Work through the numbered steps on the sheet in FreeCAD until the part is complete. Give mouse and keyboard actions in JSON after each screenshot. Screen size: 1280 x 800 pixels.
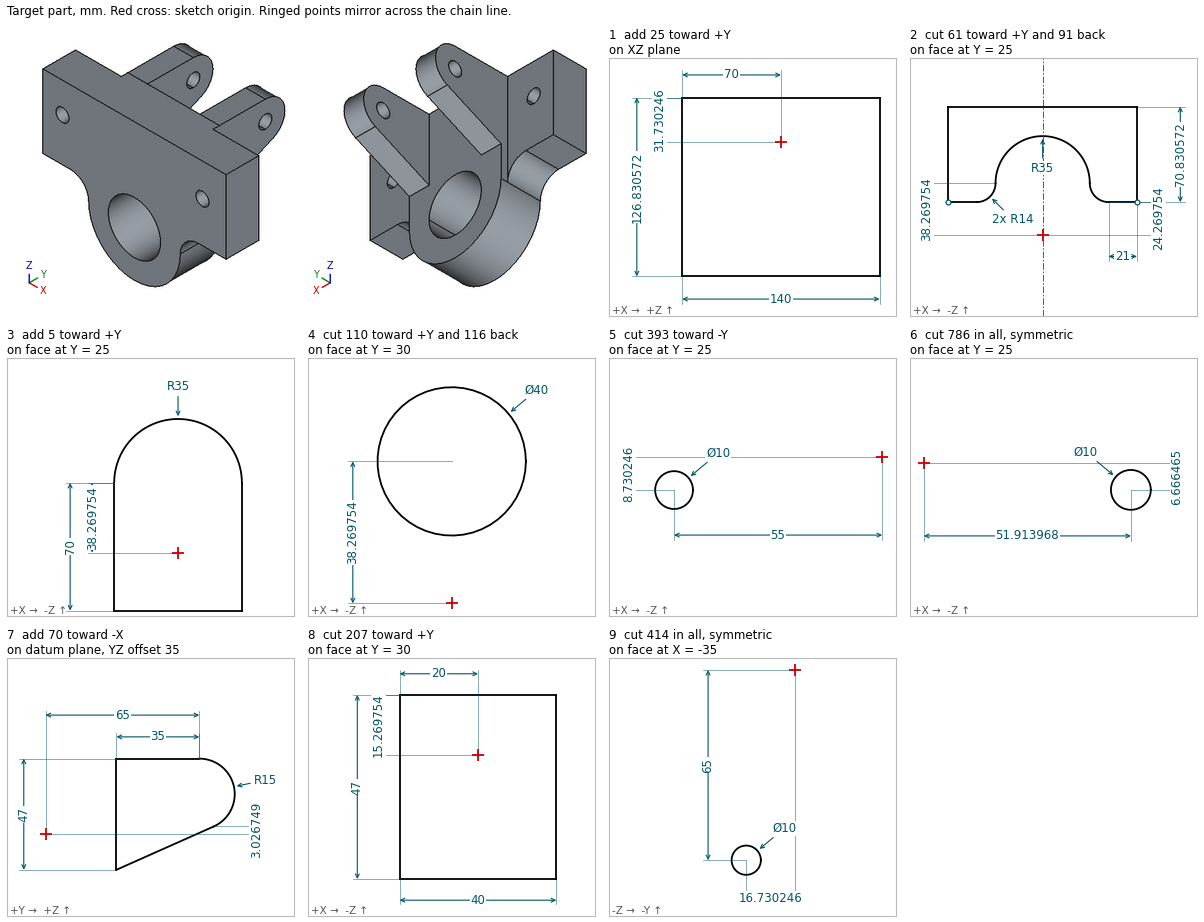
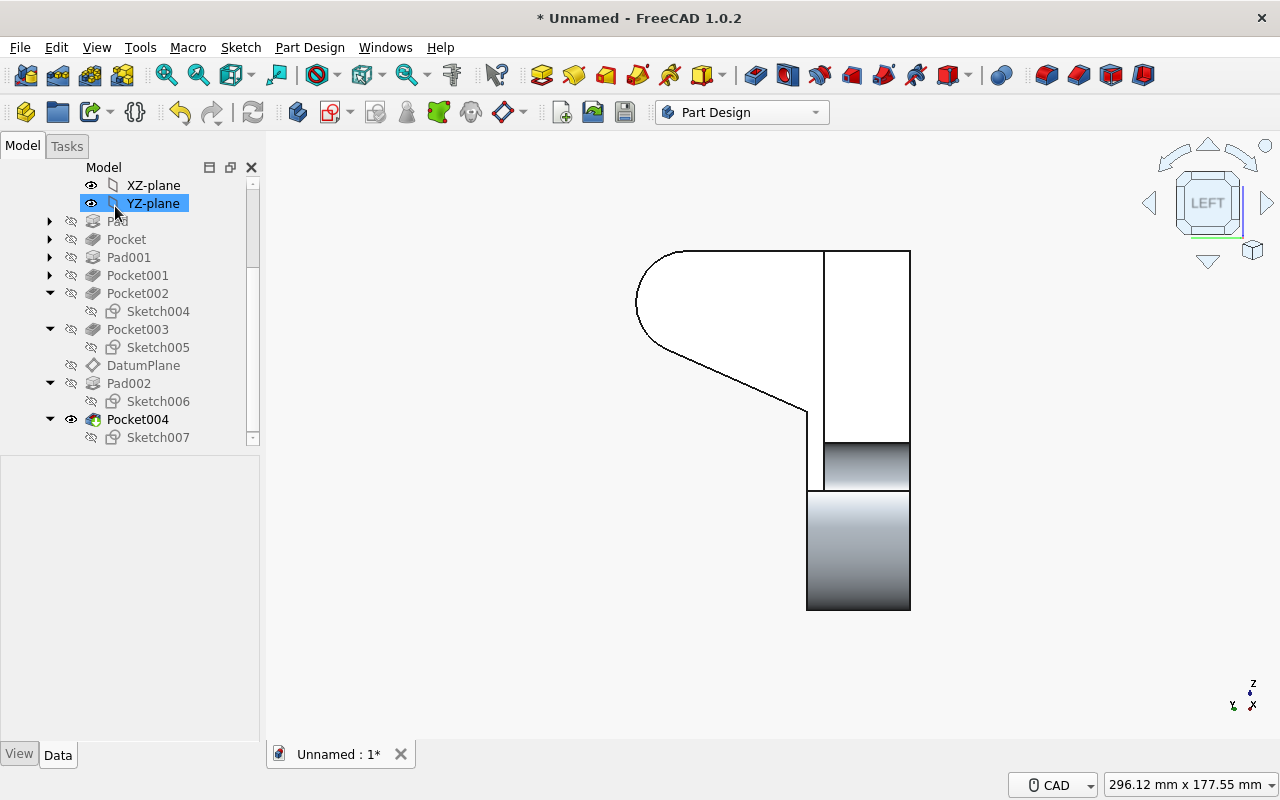
{"action": "left_click", "coordinate": [730, 301]}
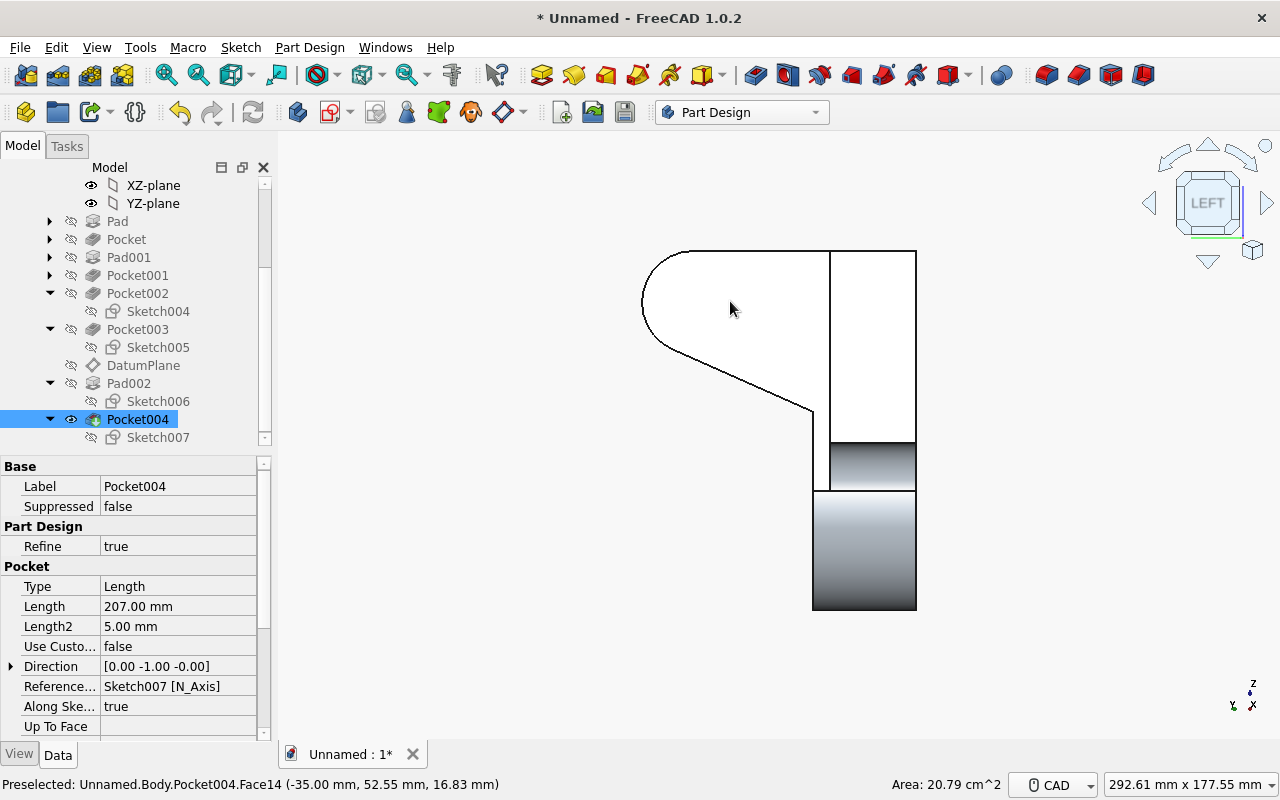
{"action": "left_click", "coordinate": [330, 112]}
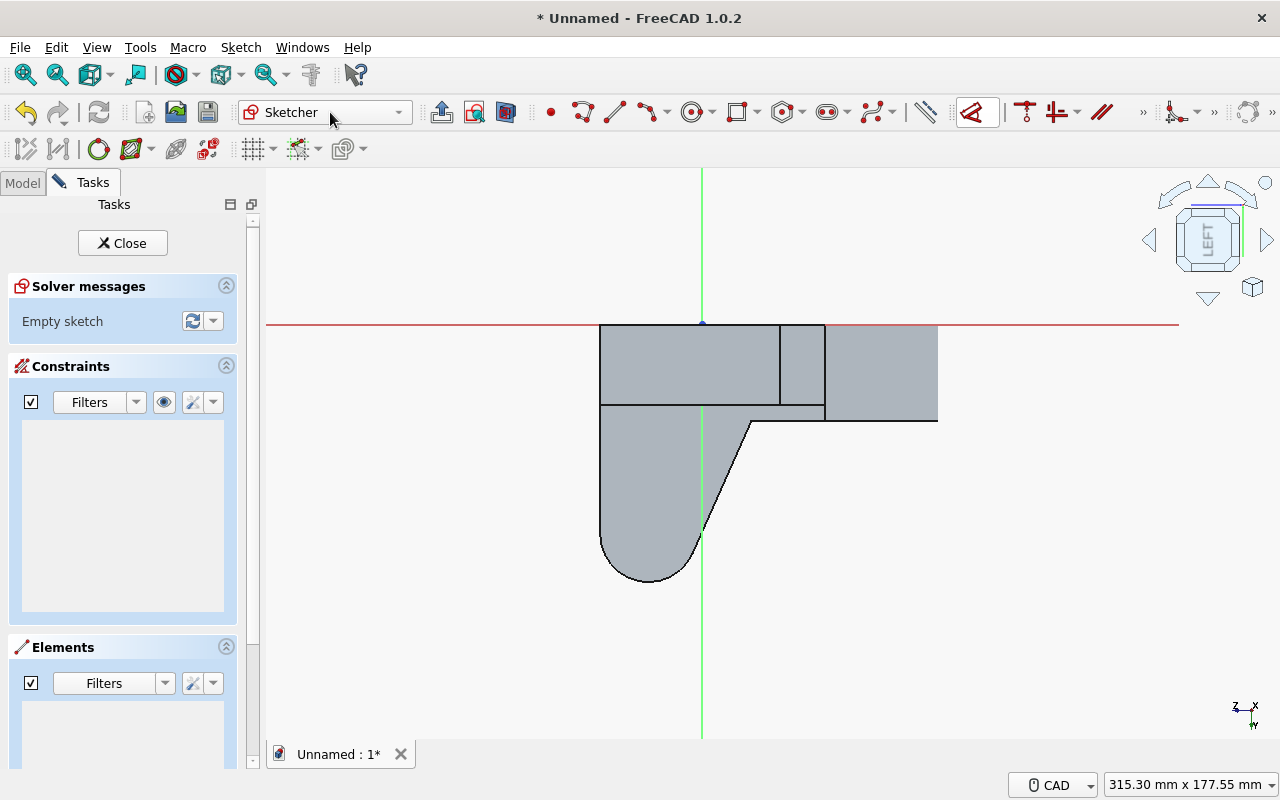
{"action": "left_click", "coordinate": [506, 112]}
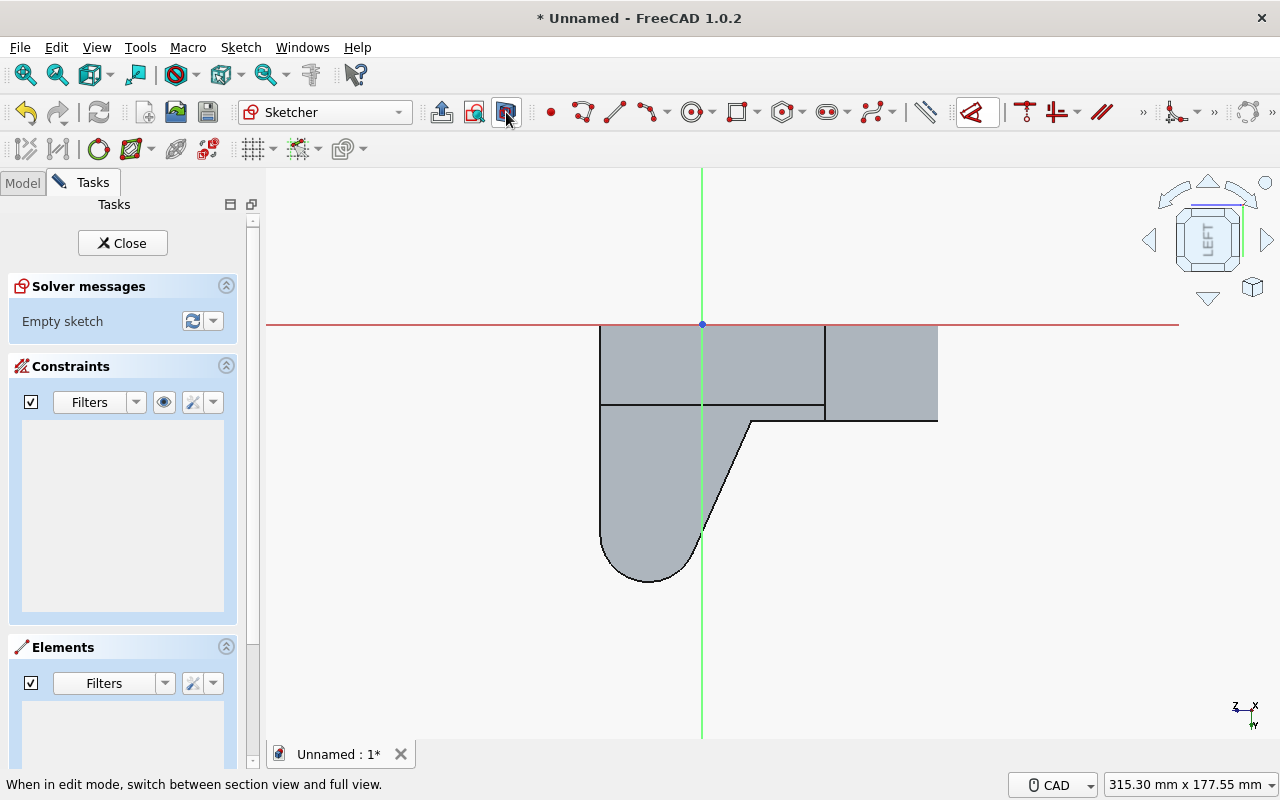
{"action": "scroll", "coordinate": [643, 542], "scroll_direction": "up", "scroll_amount": 12}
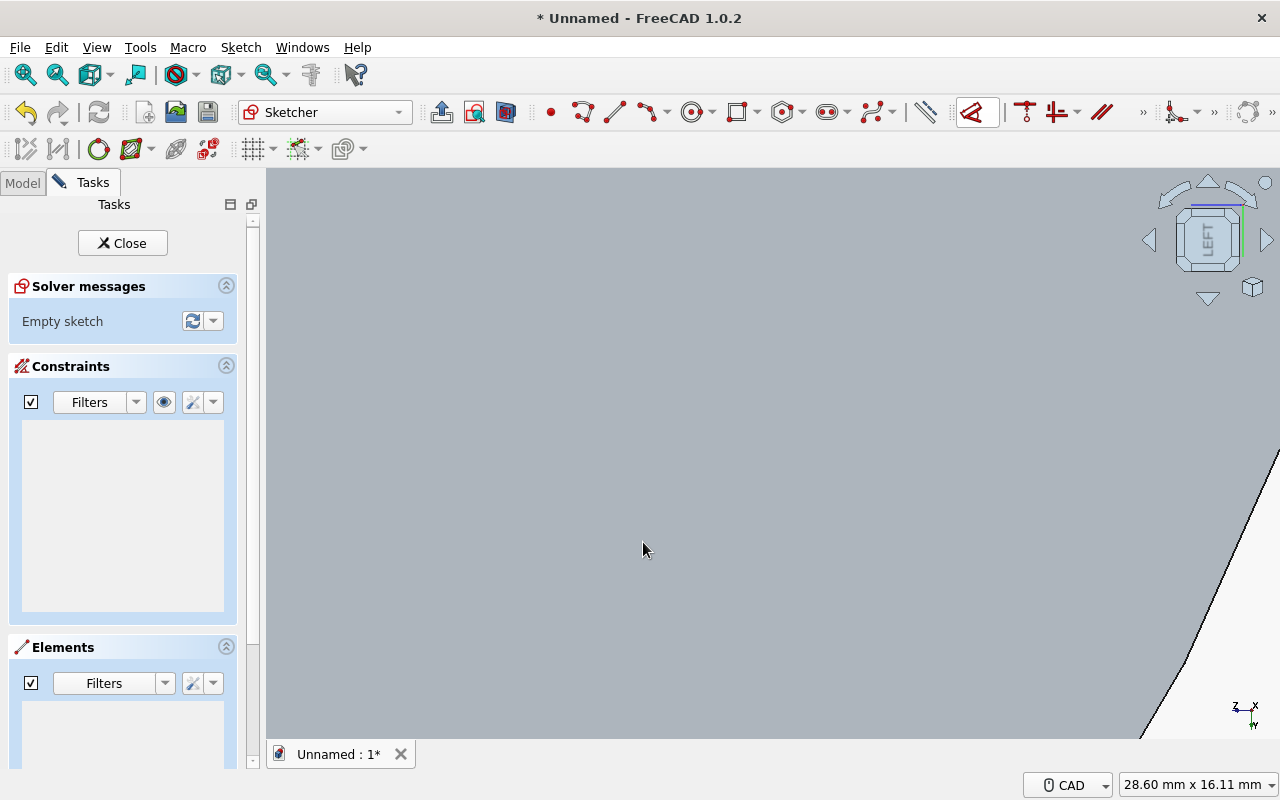
{"action": "left_click", "coordinate": [692, 112]}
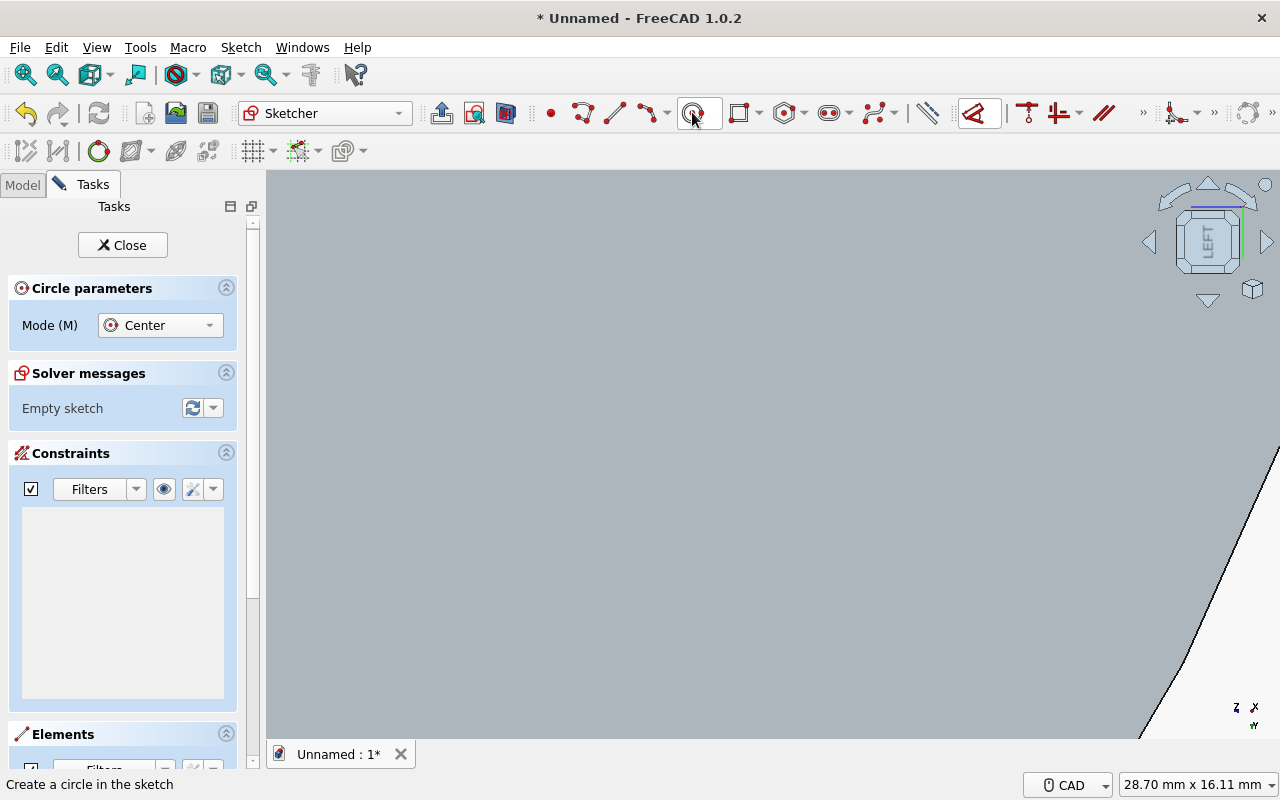
{"action": "left_click", "coordinate": [699, 447]}
{"action": "left_click", "coordinate": [824, 323]}
{"action": "key", "text": "Escape"}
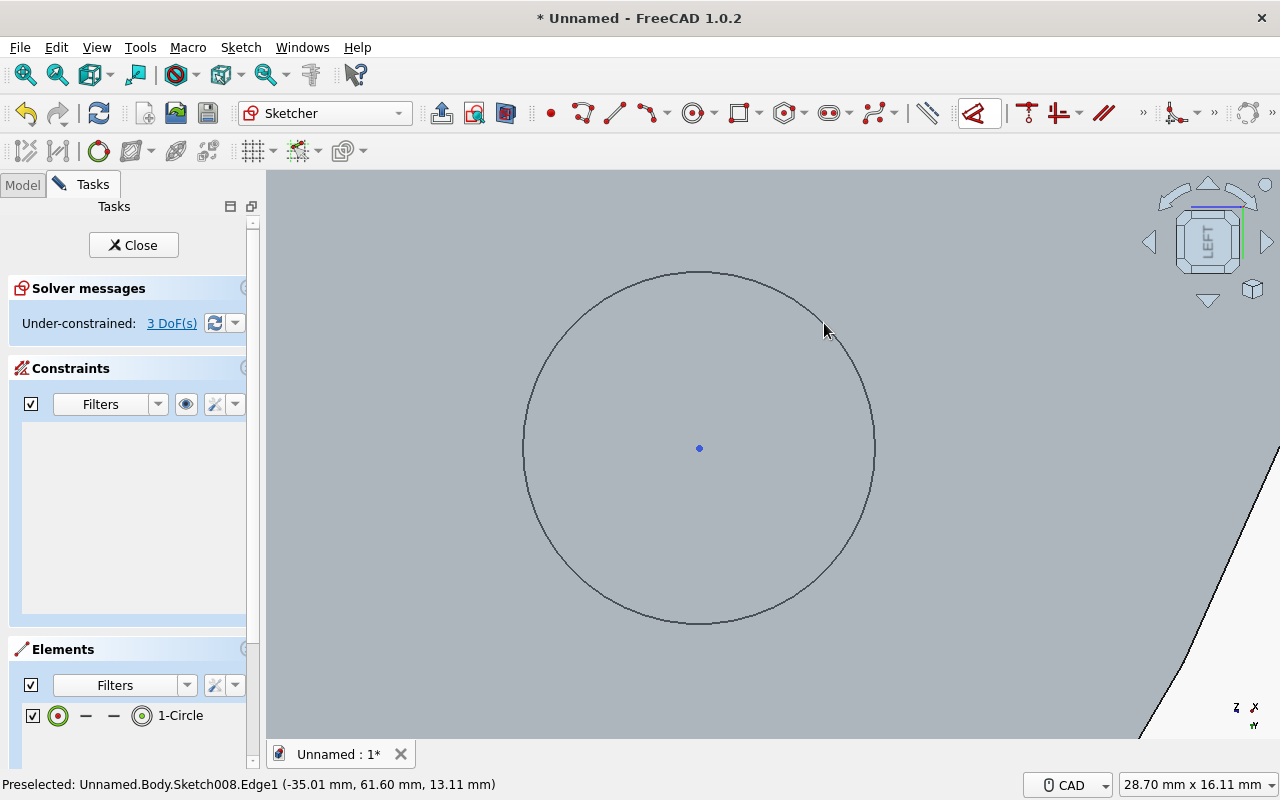
{"action": "left_click", "coordinate": [823, 323]}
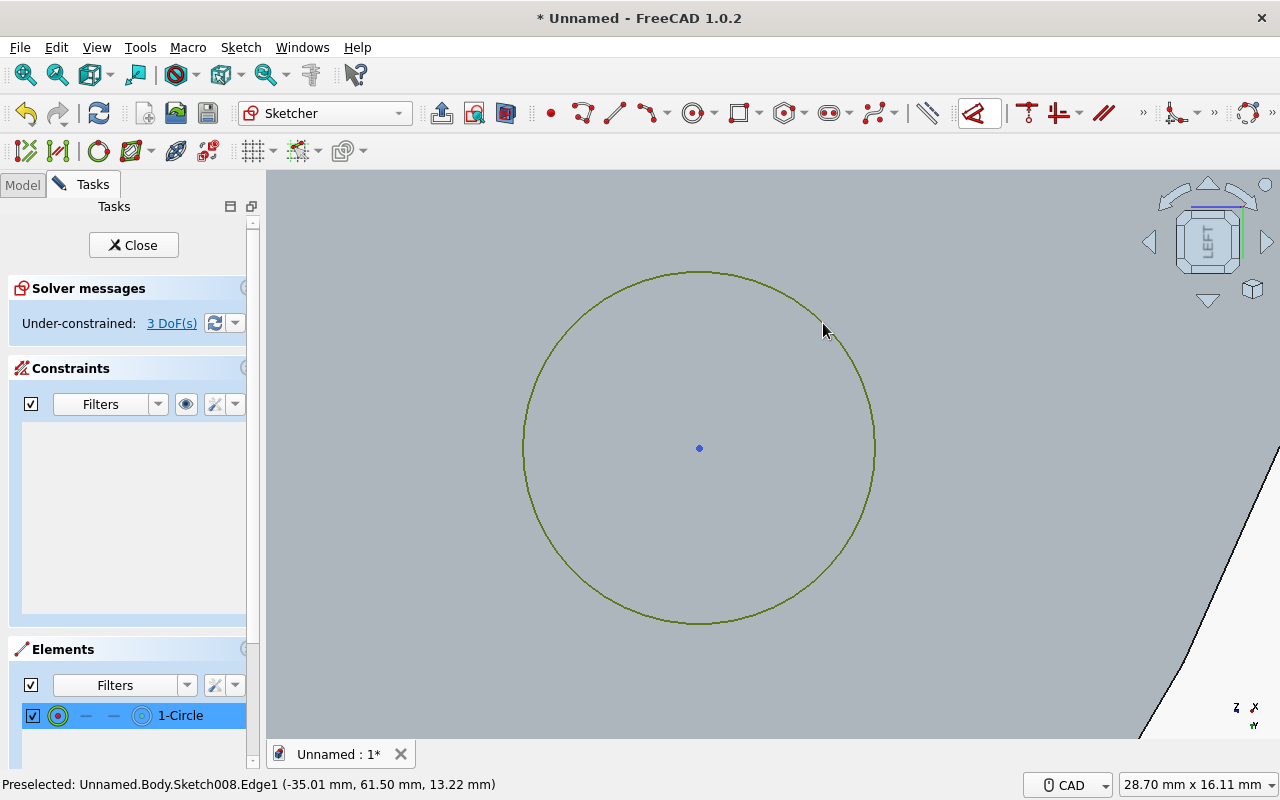
{"action": "left_click", "coordinate": [996, 114]}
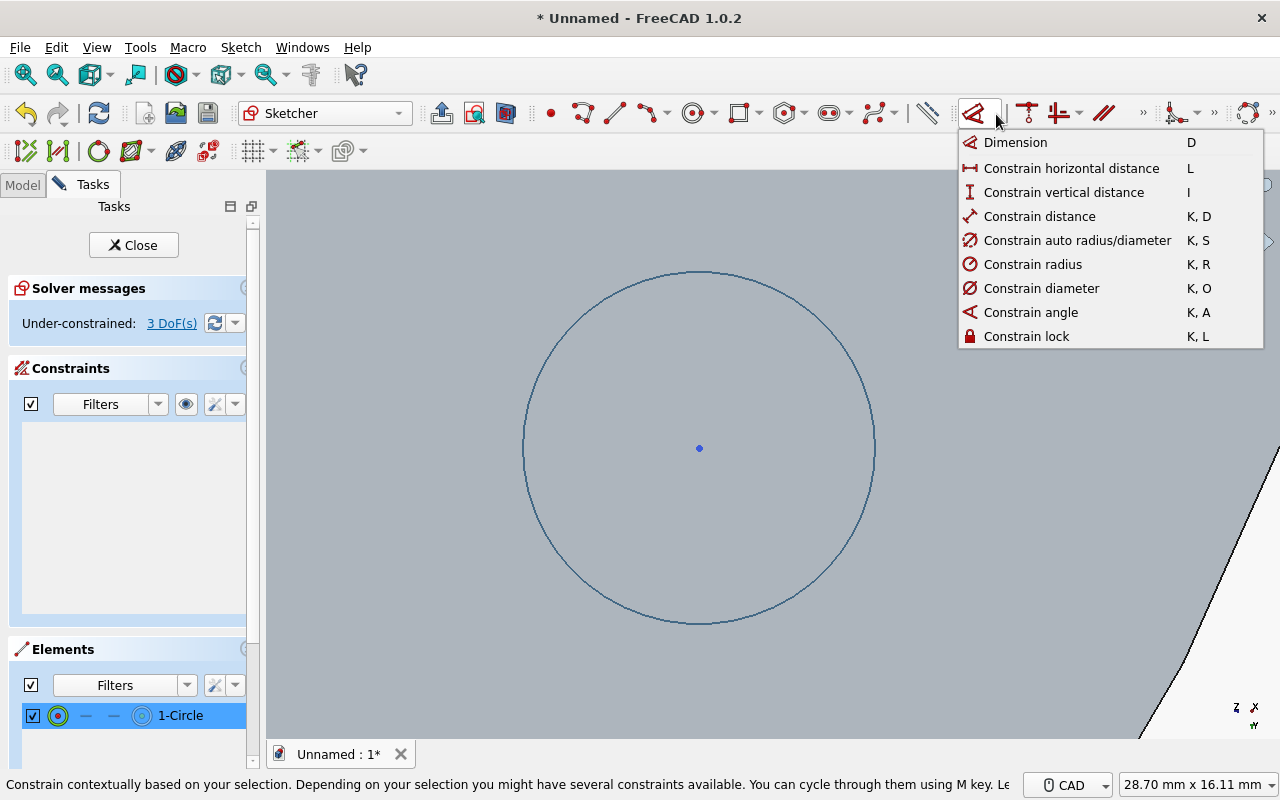
{"action": "left_click", "coordinate": [1111, 288]}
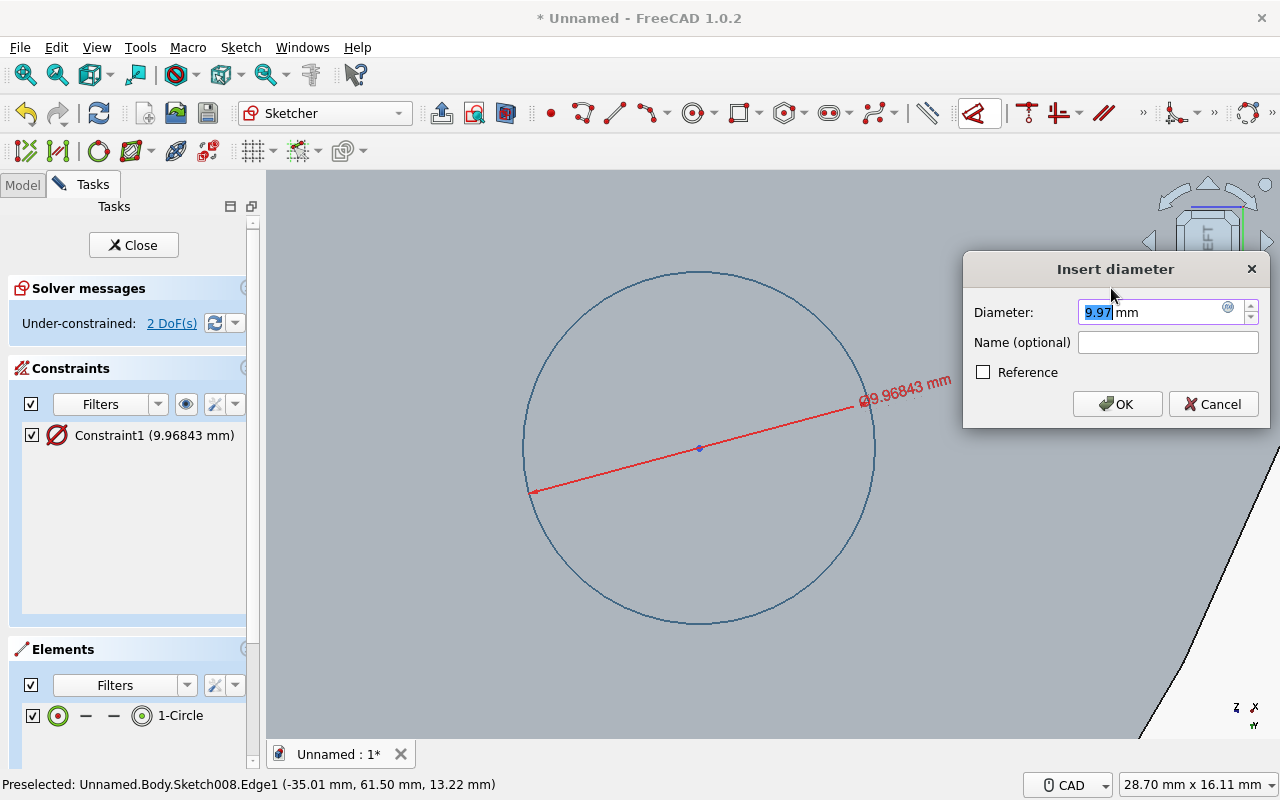
{"action": "type", "text": "10"}
{"action": "key", "text": "Return"}